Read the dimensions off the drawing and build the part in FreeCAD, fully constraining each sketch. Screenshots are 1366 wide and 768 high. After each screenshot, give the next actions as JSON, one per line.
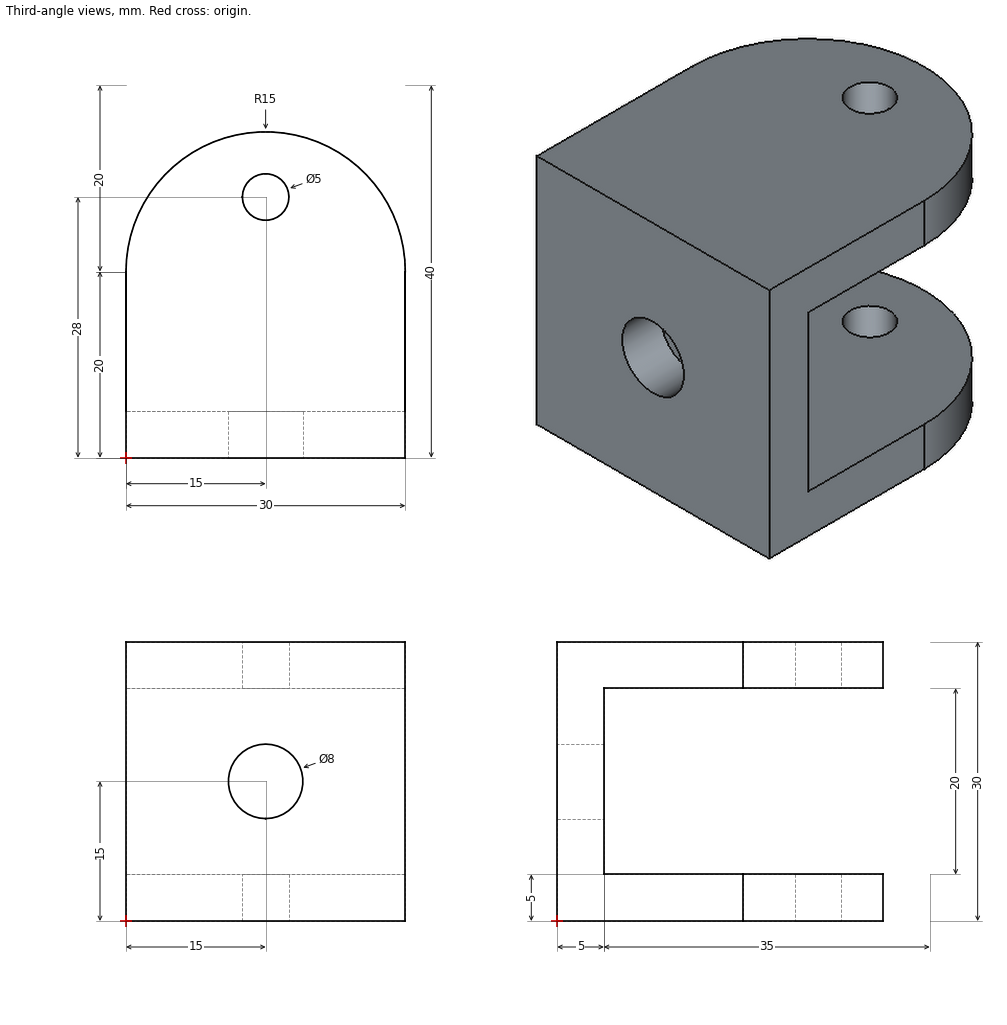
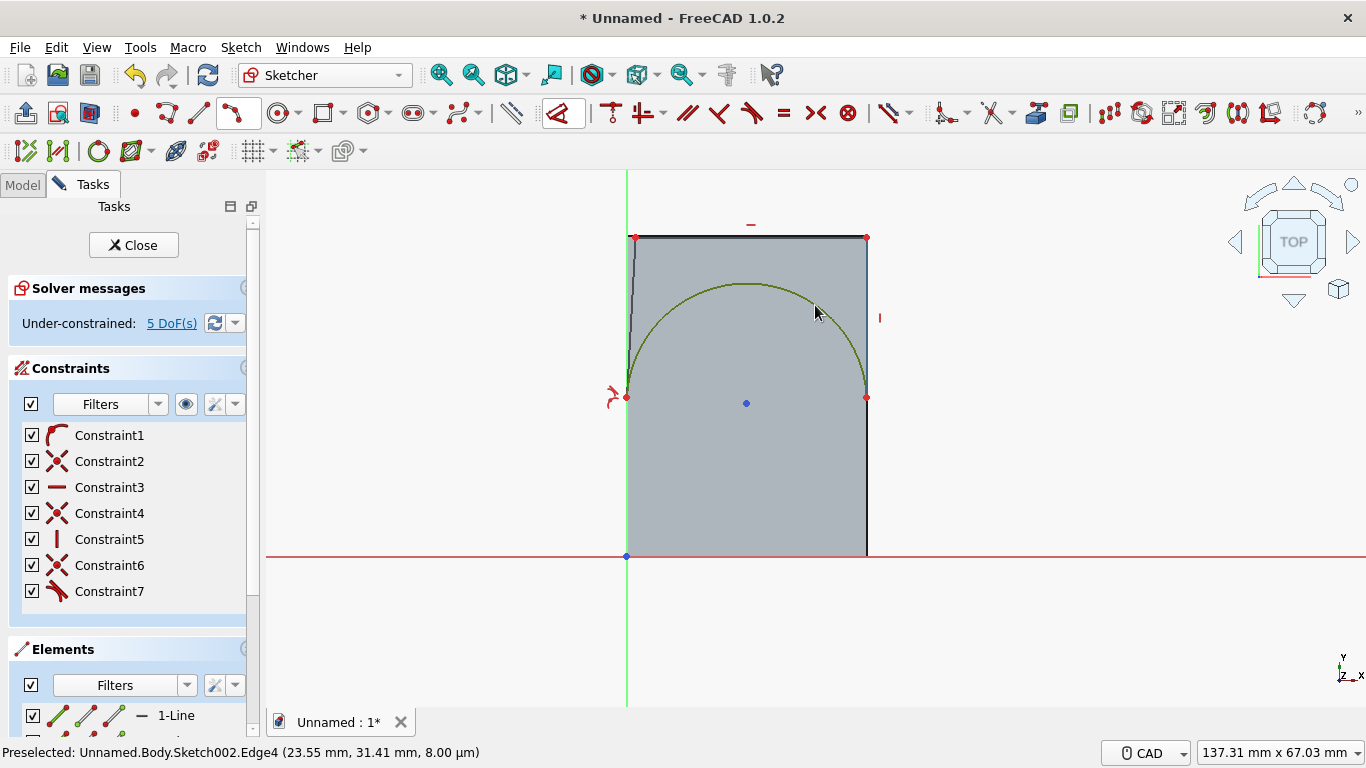
{"action": "left_click", "coordinate": [752, 114]}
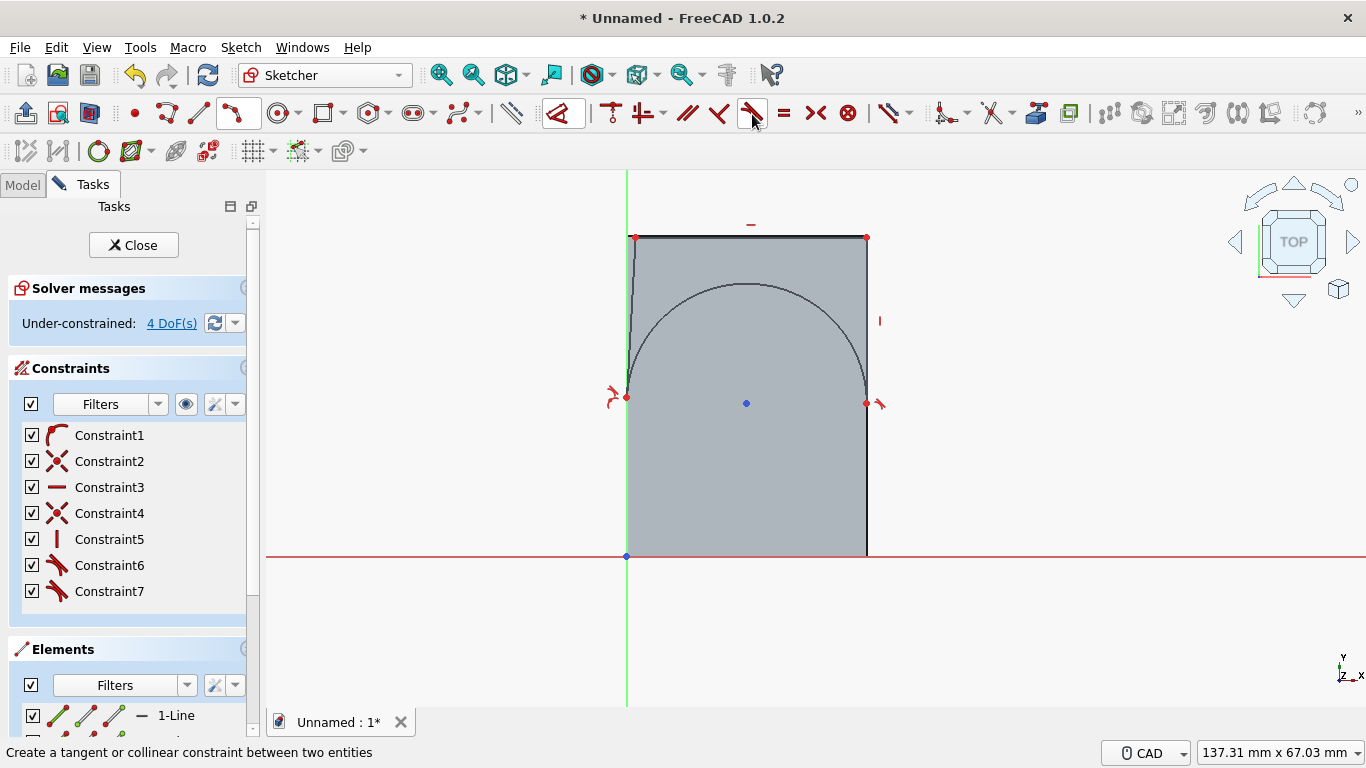
{"action": "scroll", "coordinate": [630, 349], "scroll_direction": "up", "scroll_amount": 3}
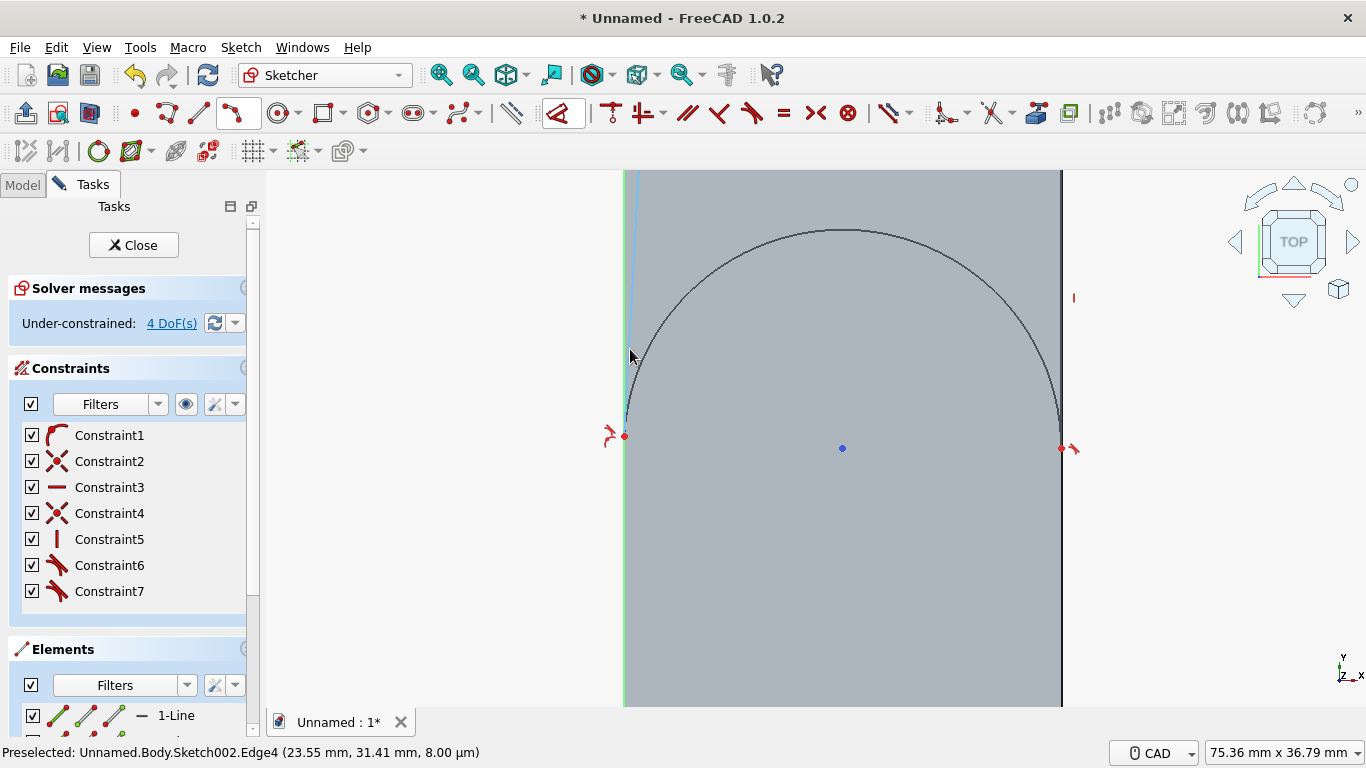
{"action": "left_click", "coordinate": [629, 349]}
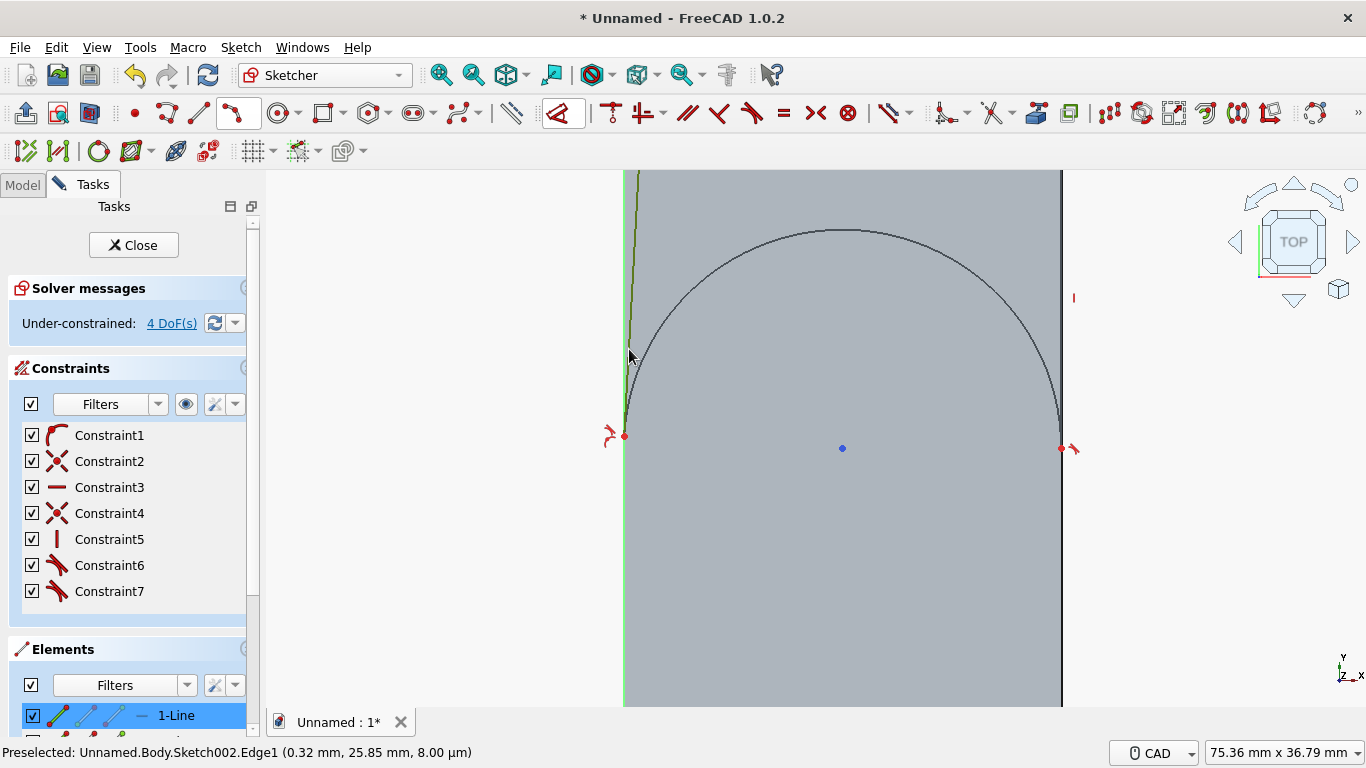
{"action": "left_click", "coordinate": [666, 114]}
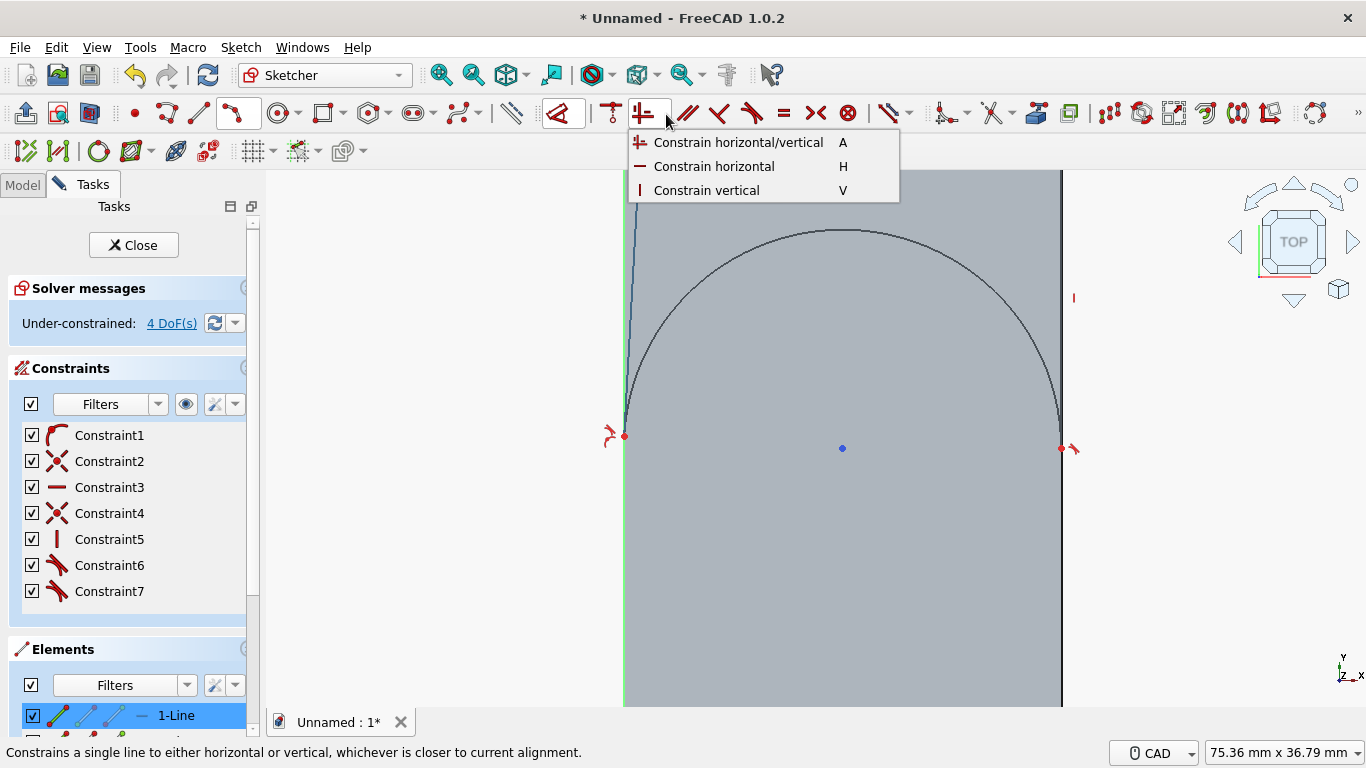
{"action": "left_click", "coordinate": [764, 190]}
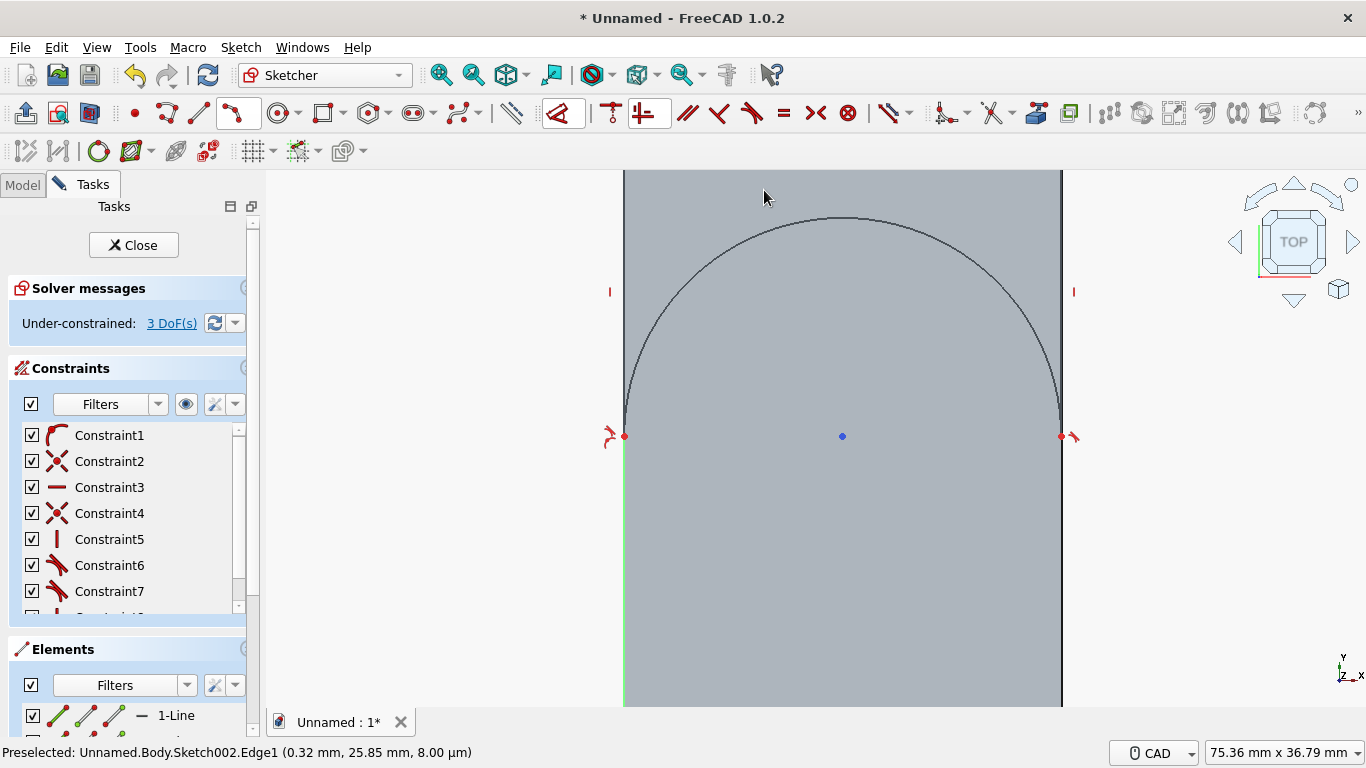
{"action": "left_click", "coordinate": [971, 260]}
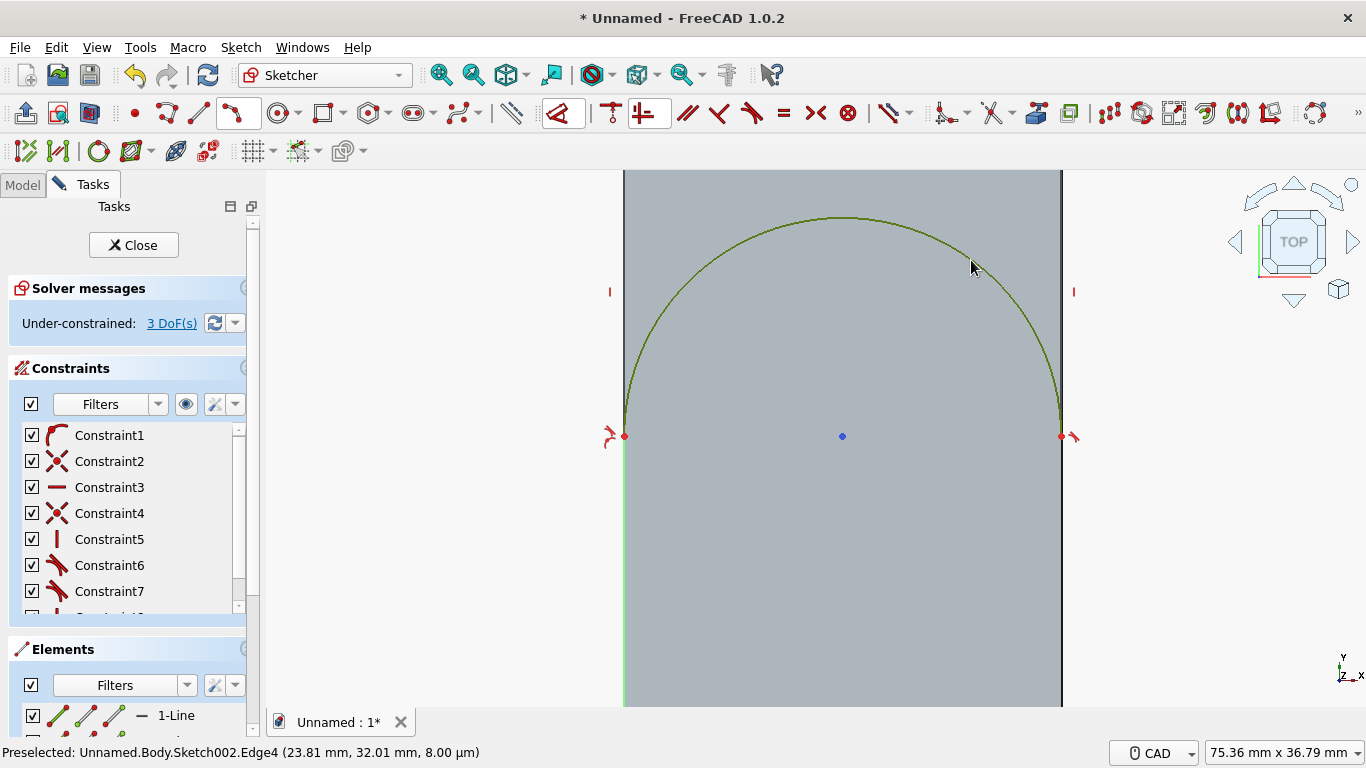
{"action": "left_click", "coordinate": [580, 114]}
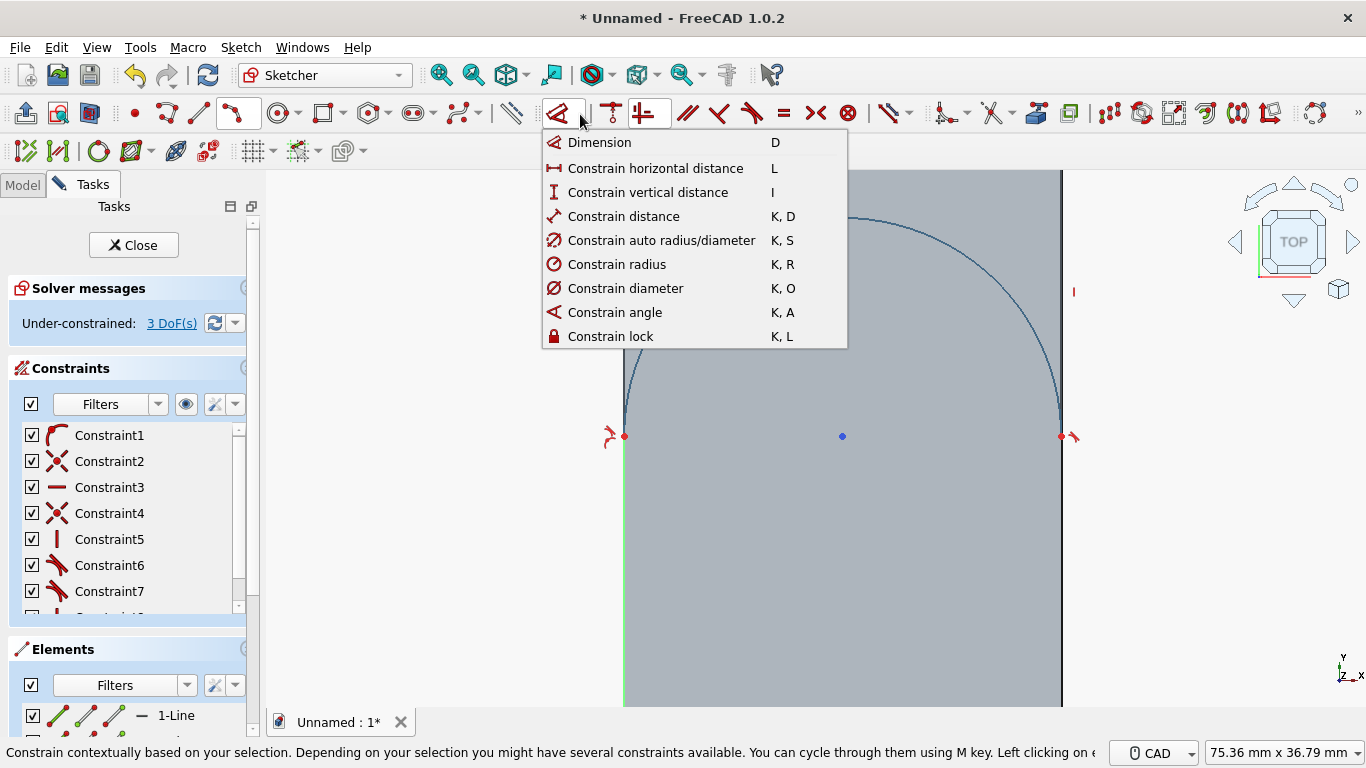
{"action": "left_click", "coordinate": [695, 264]}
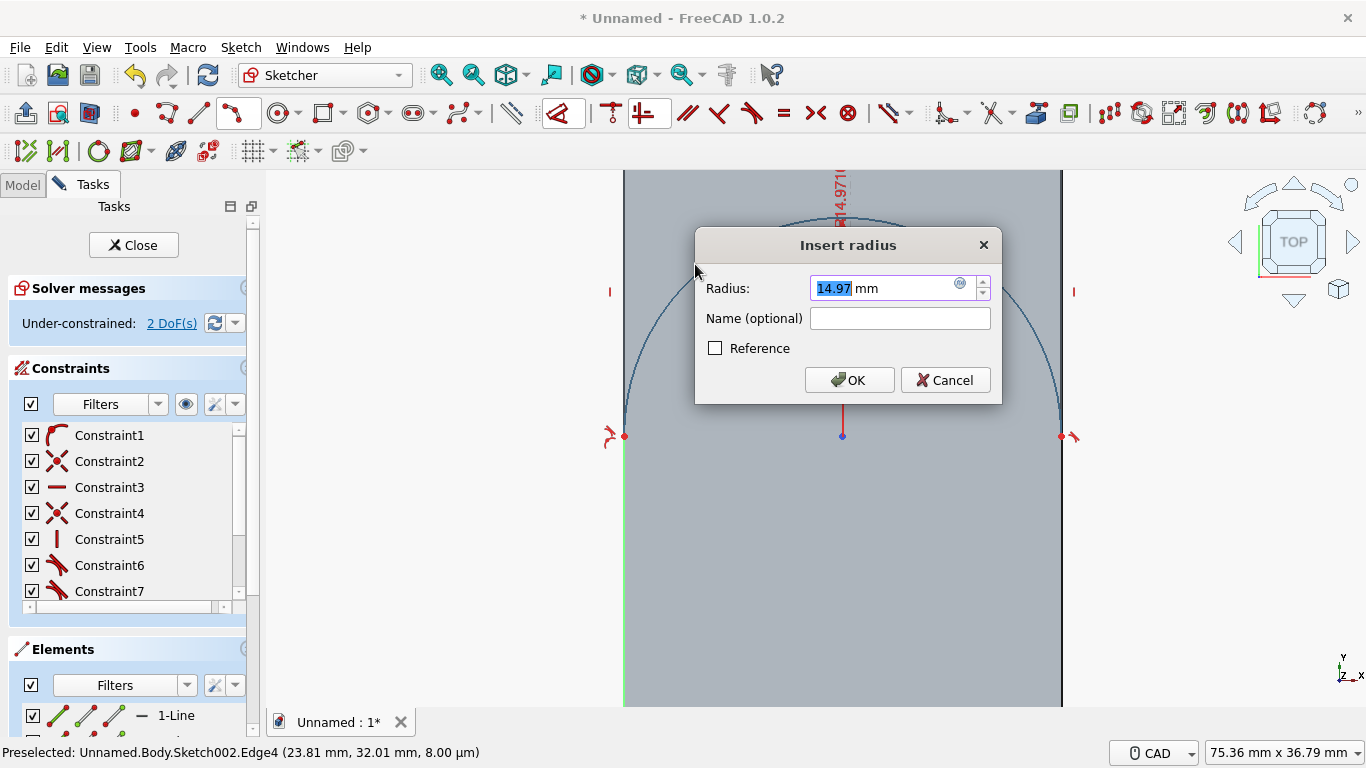
{"action": "type", "text": "15"}
{"action": "key", "text": "Return"}